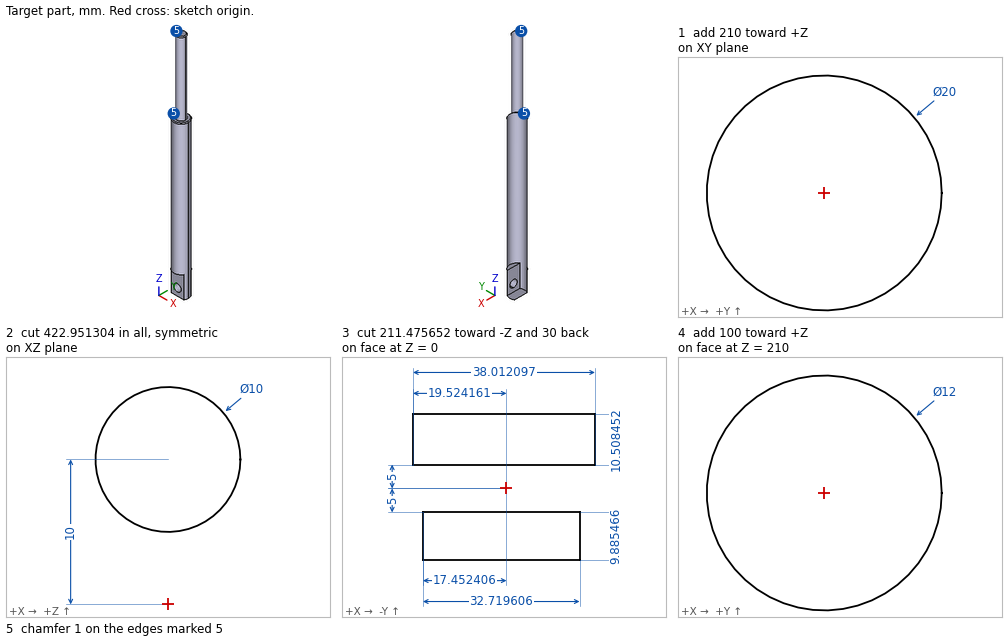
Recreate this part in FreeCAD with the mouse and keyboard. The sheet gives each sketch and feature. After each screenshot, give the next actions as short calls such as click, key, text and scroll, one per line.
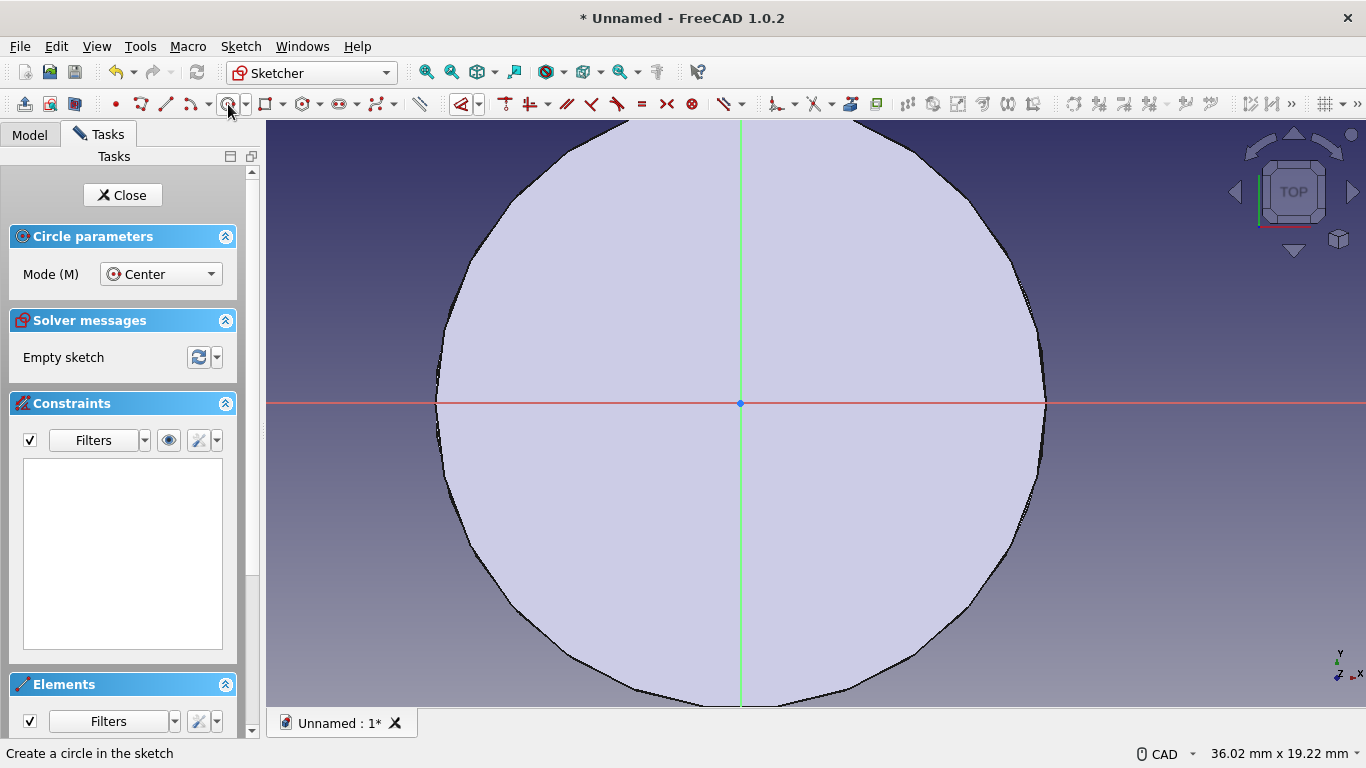
click(741, 403)
move(870, 274)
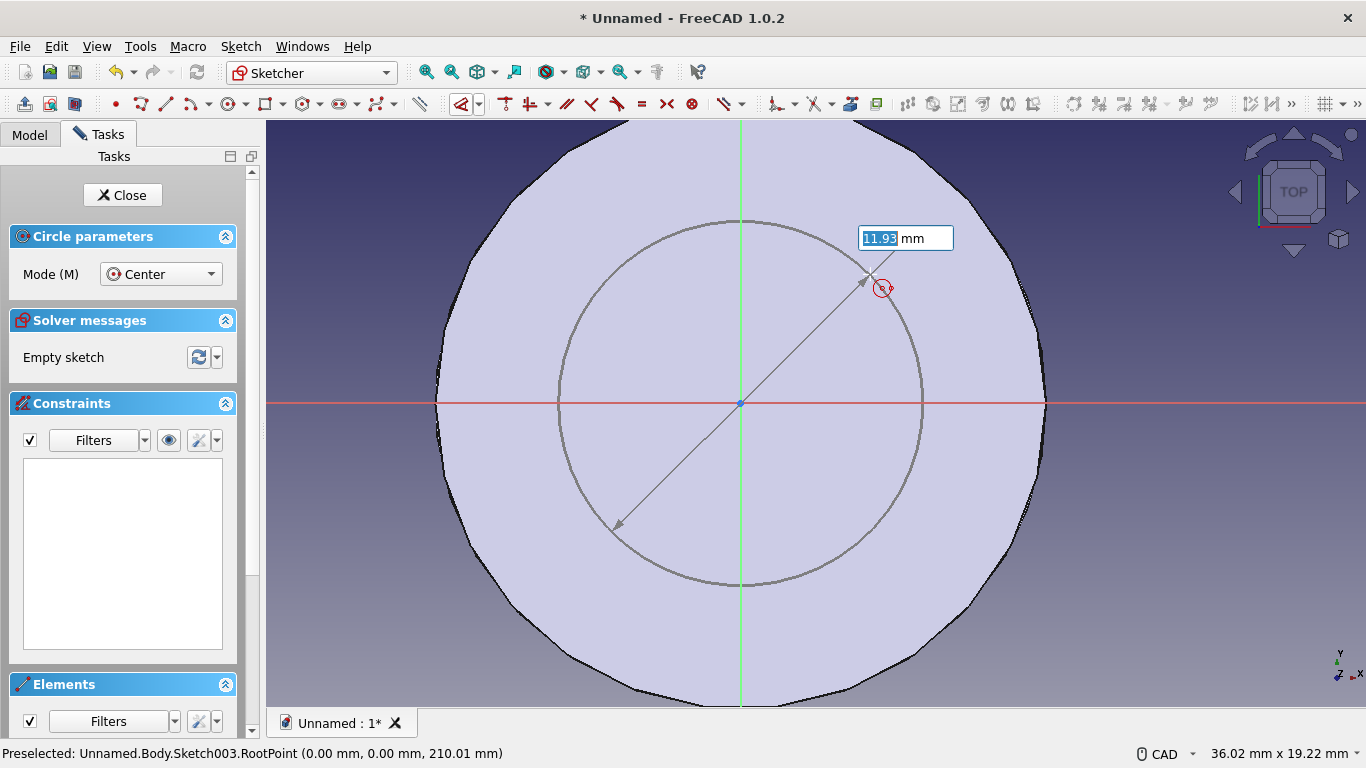
text(12)
key(Return)
key(Escape)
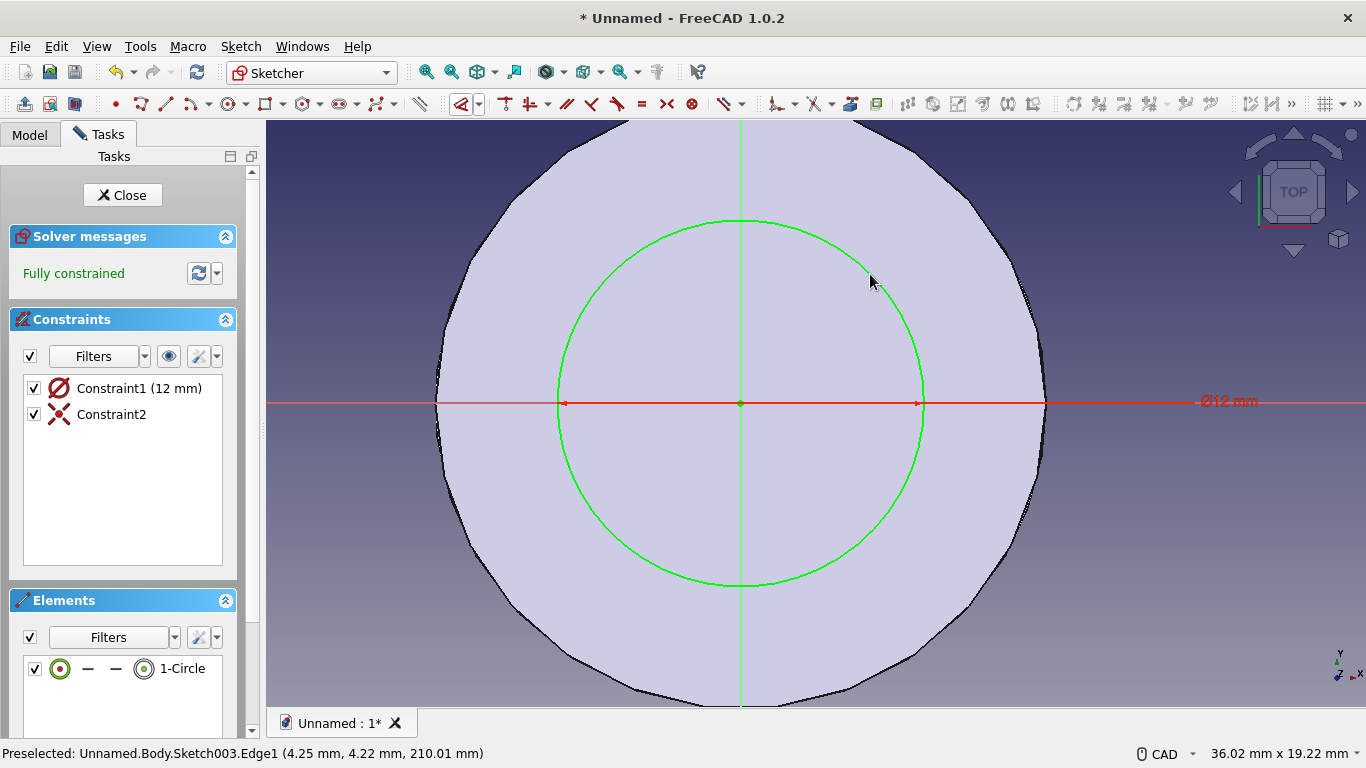
click(123, 195)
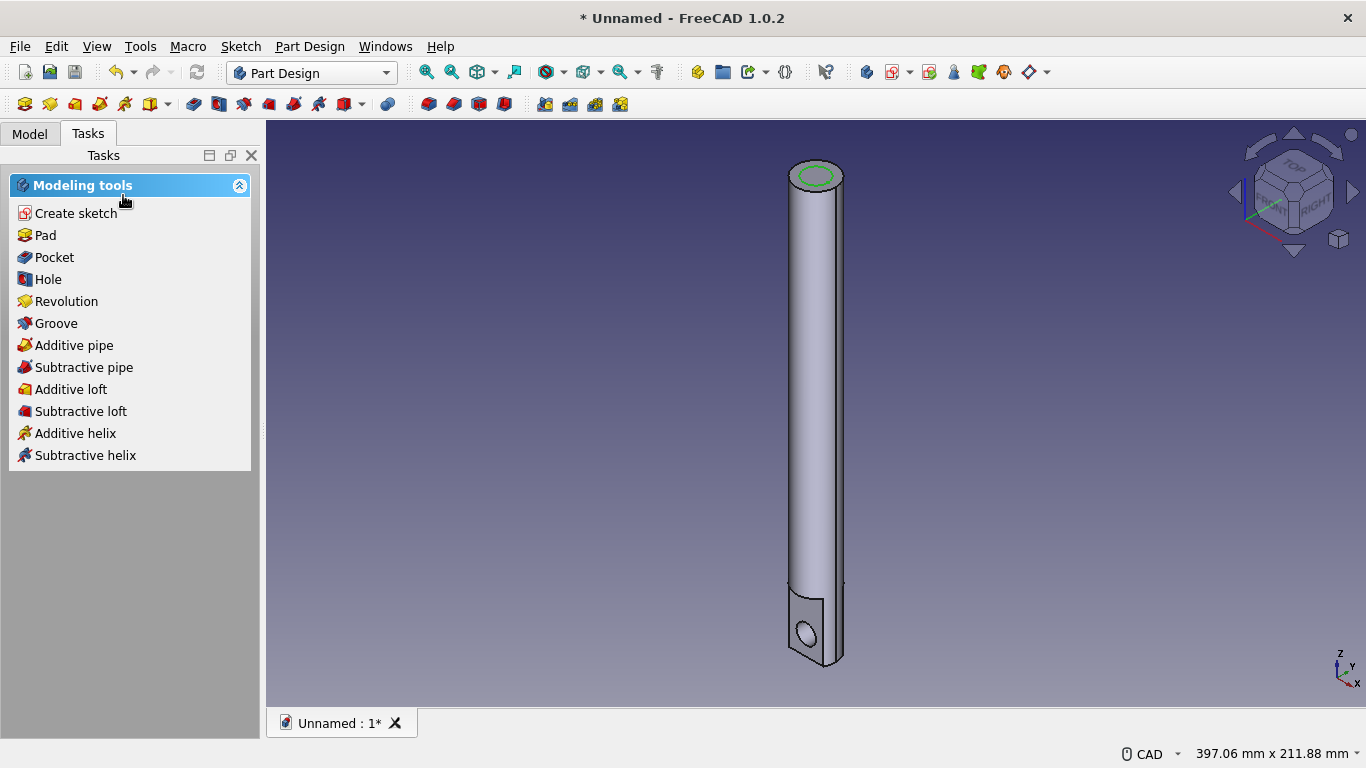
click(25, 104)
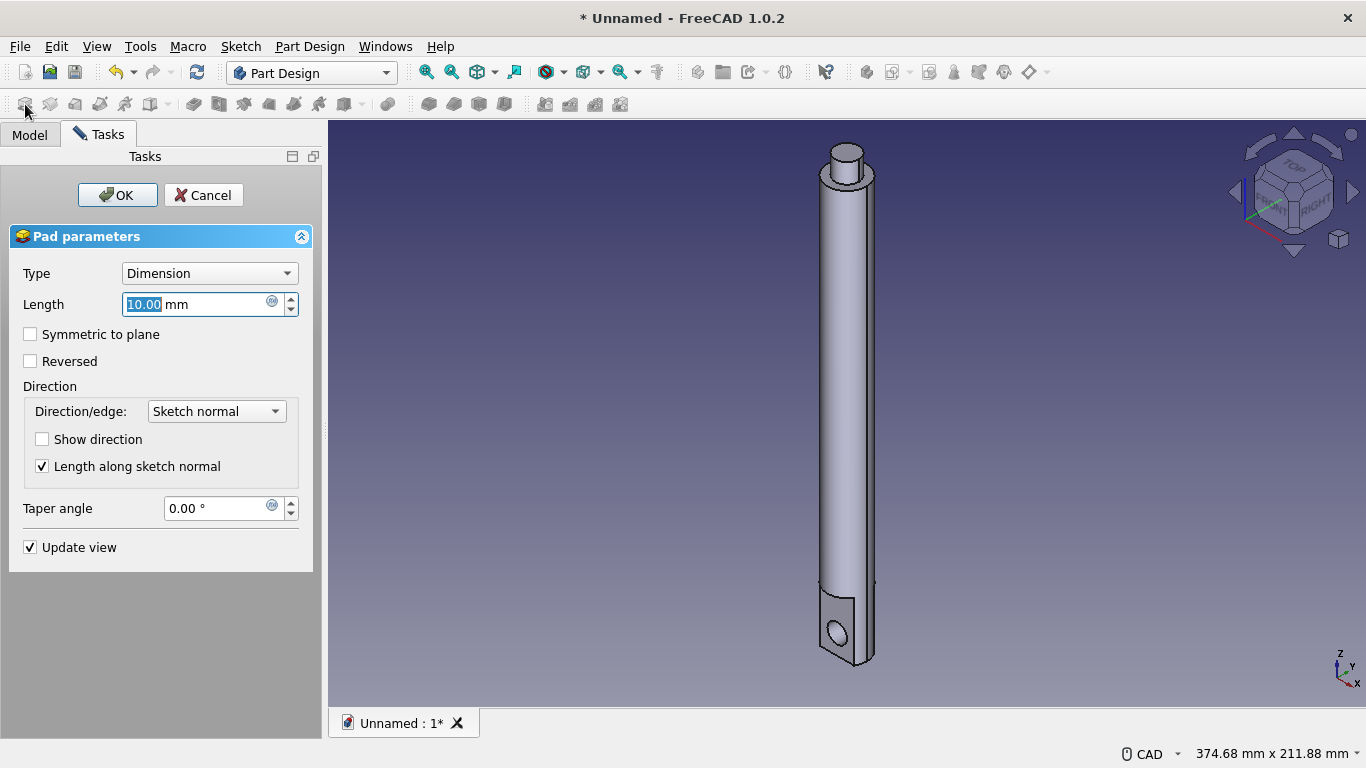
text(100)
key(Tab)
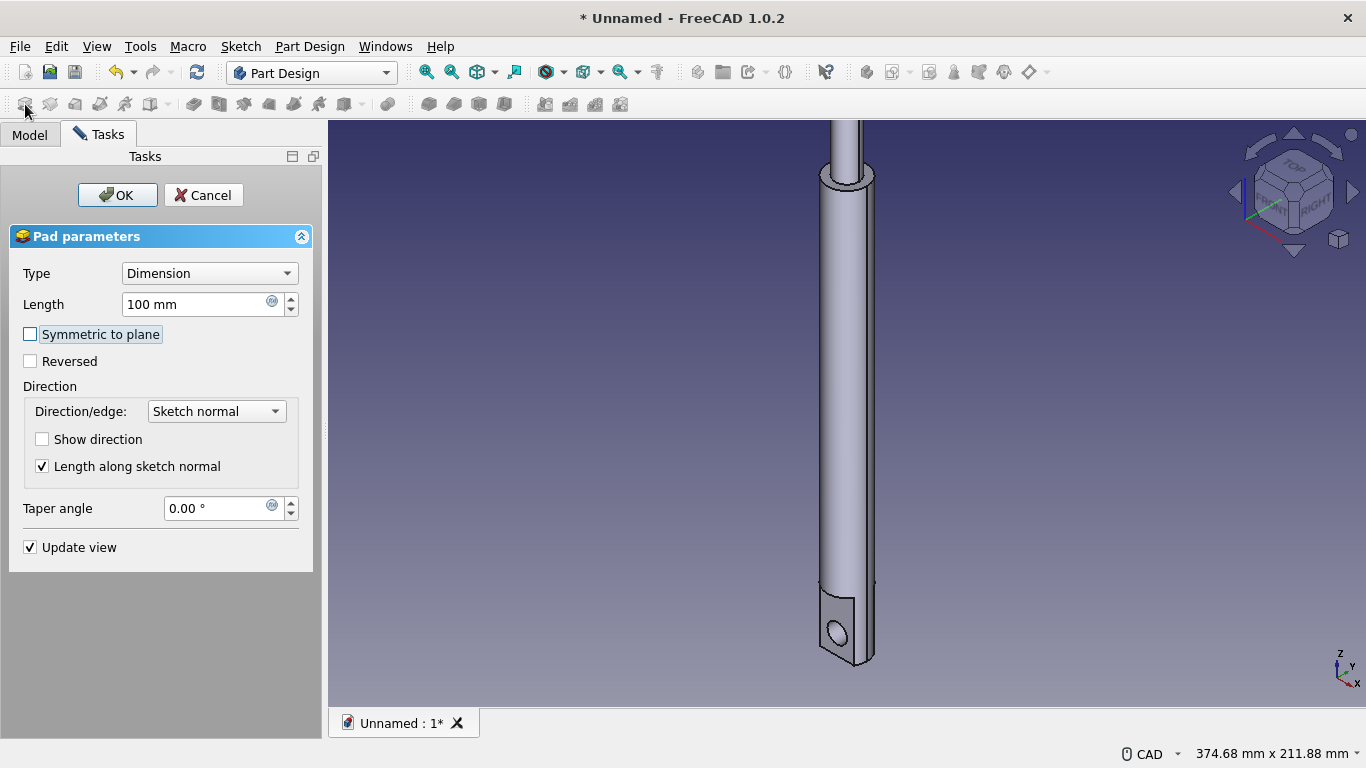
click(118, 195)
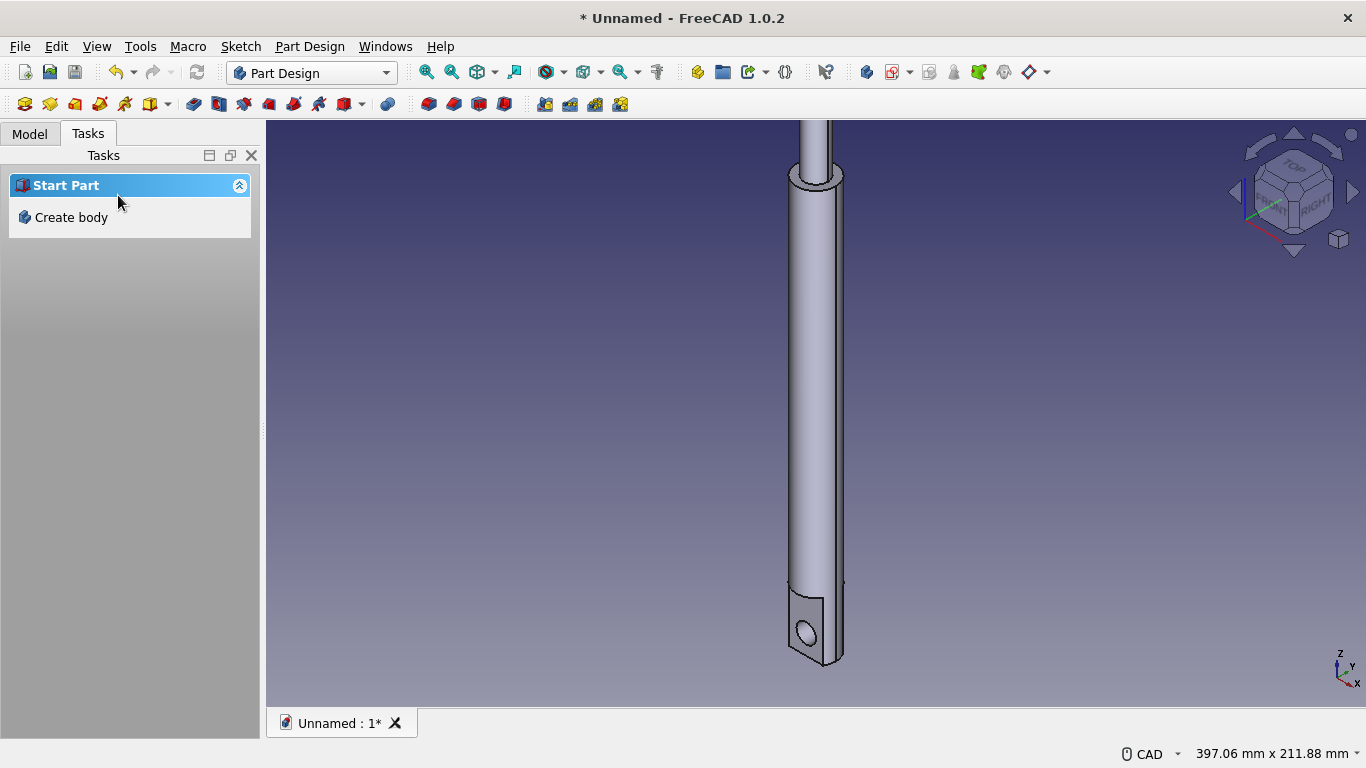
click(427, 72)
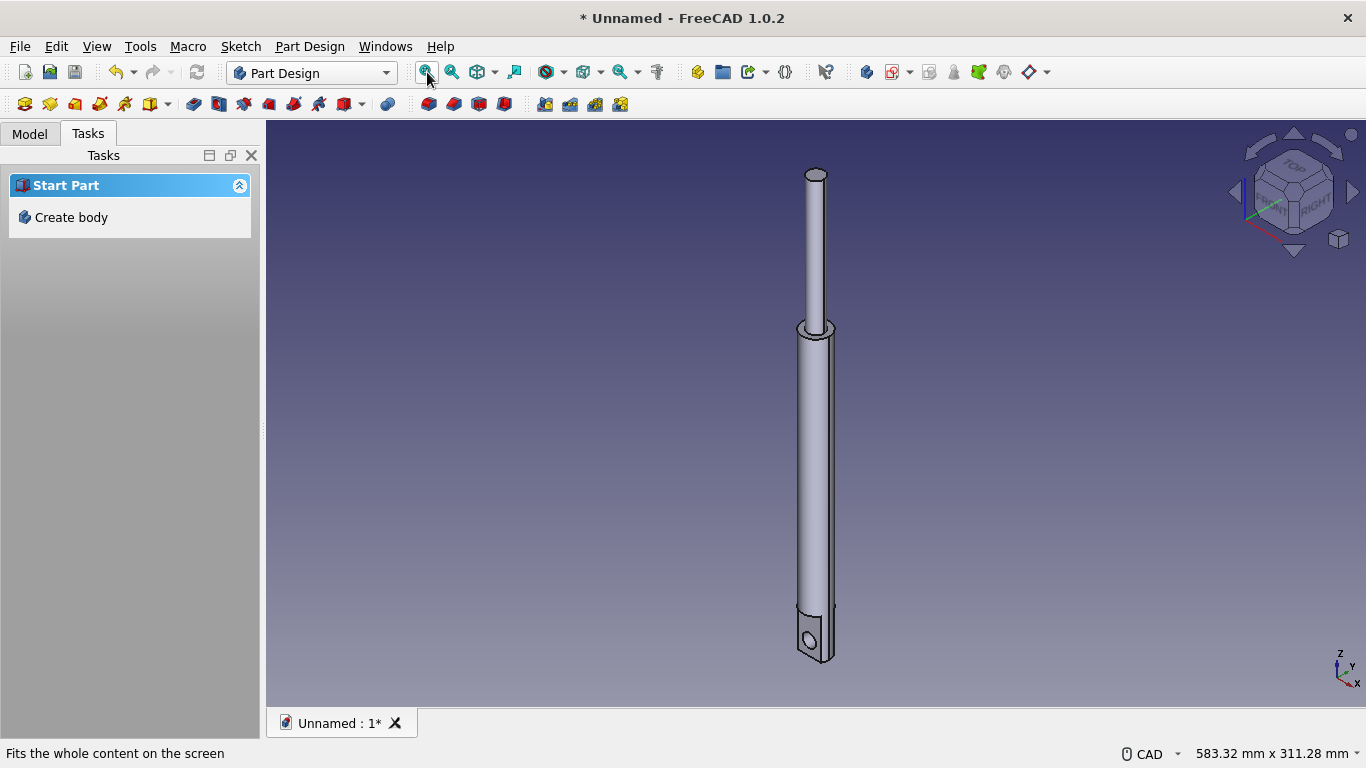
click(797, 326)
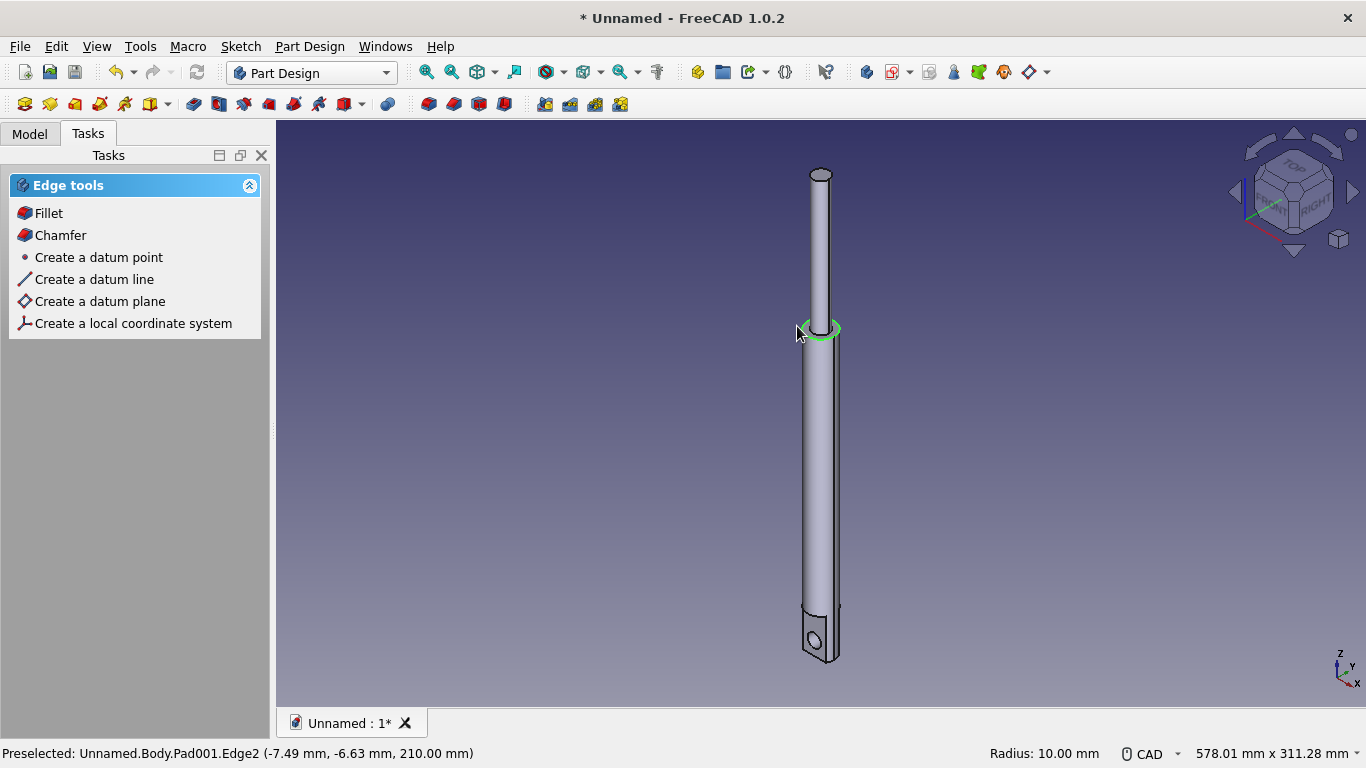
click(813, 169, ctrl)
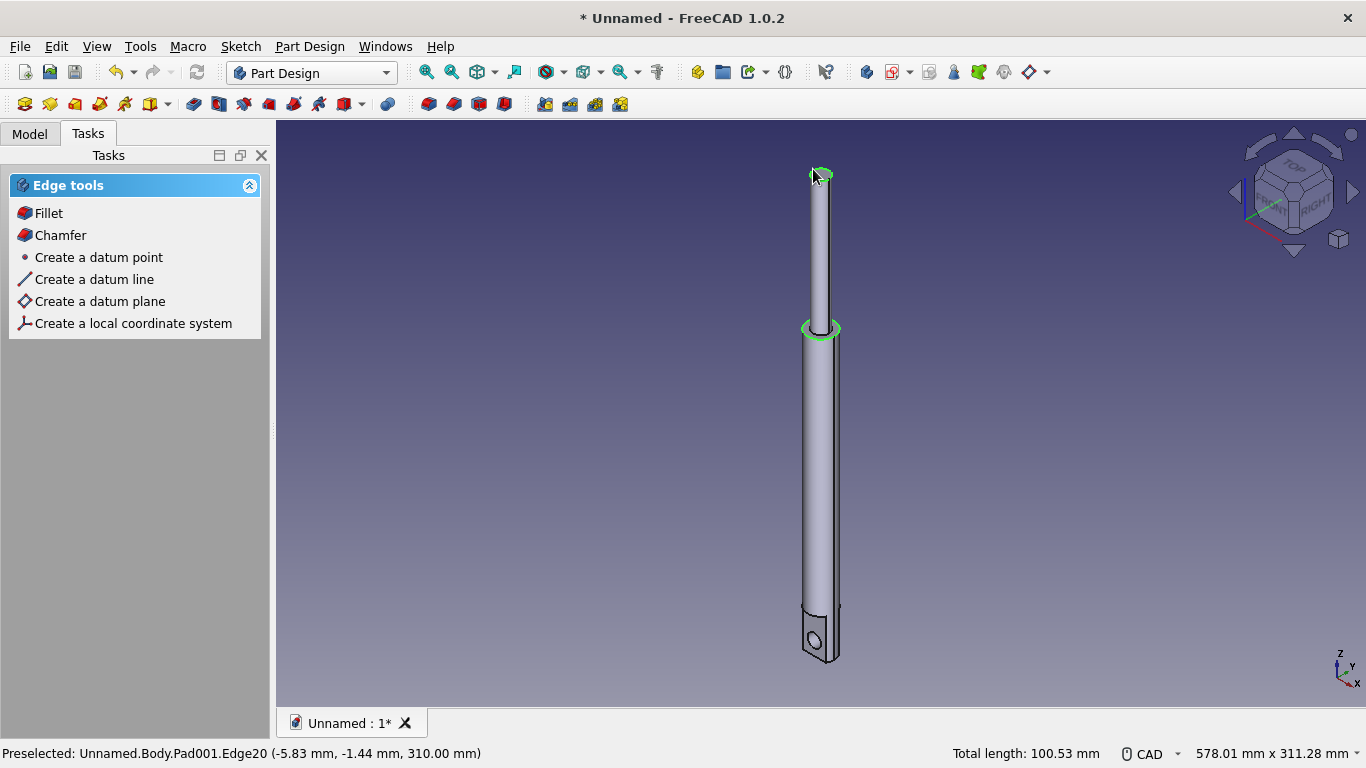
click(454, 104)